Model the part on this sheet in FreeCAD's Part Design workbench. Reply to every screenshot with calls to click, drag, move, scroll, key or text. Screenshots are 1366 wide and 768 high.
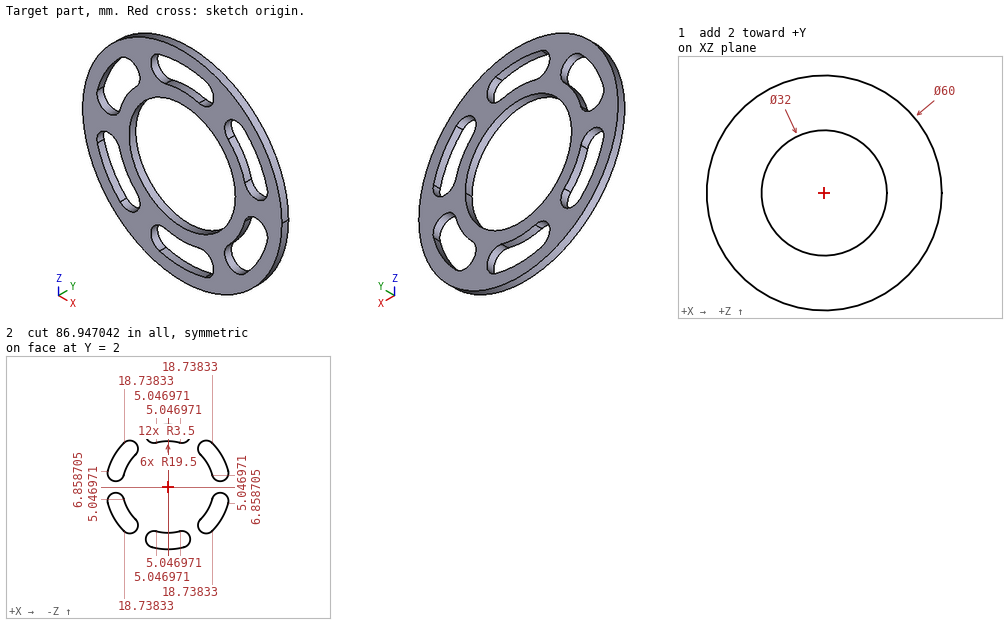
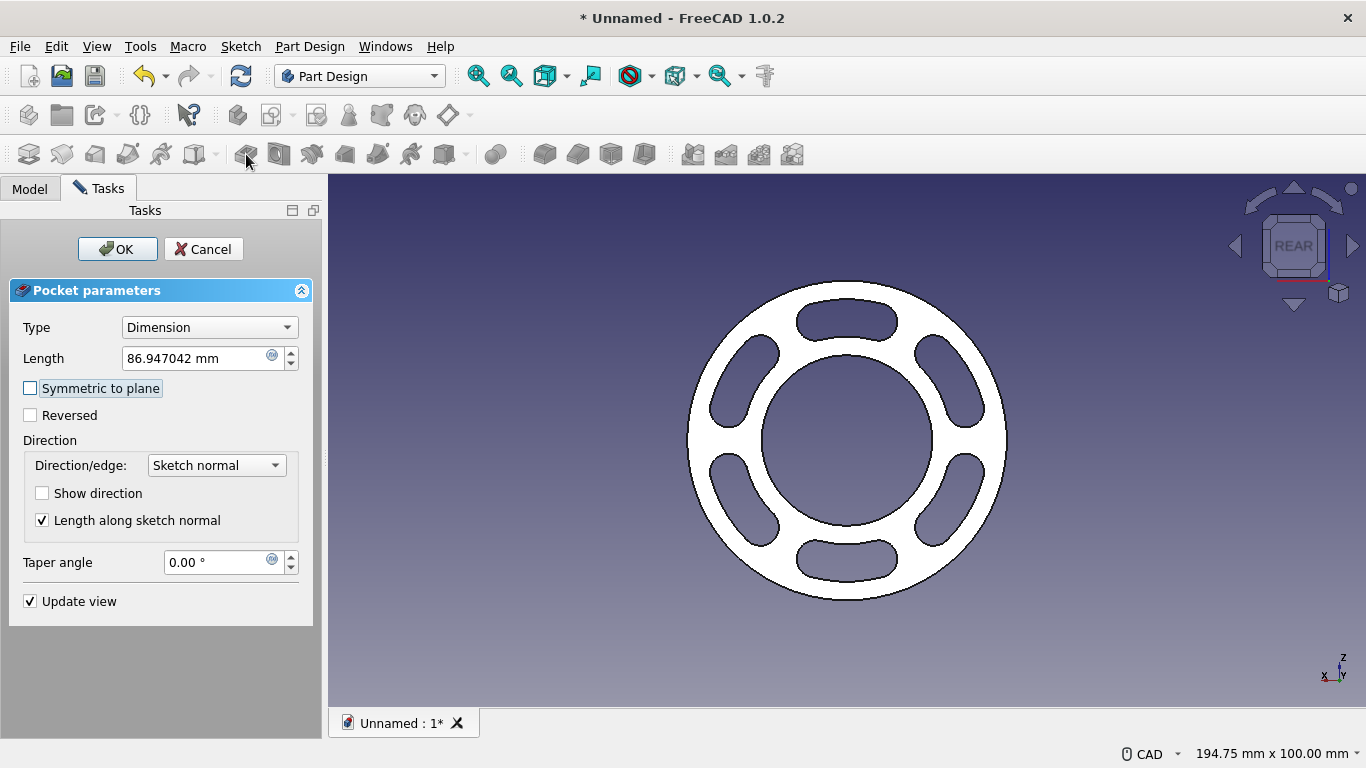
click(31, 388)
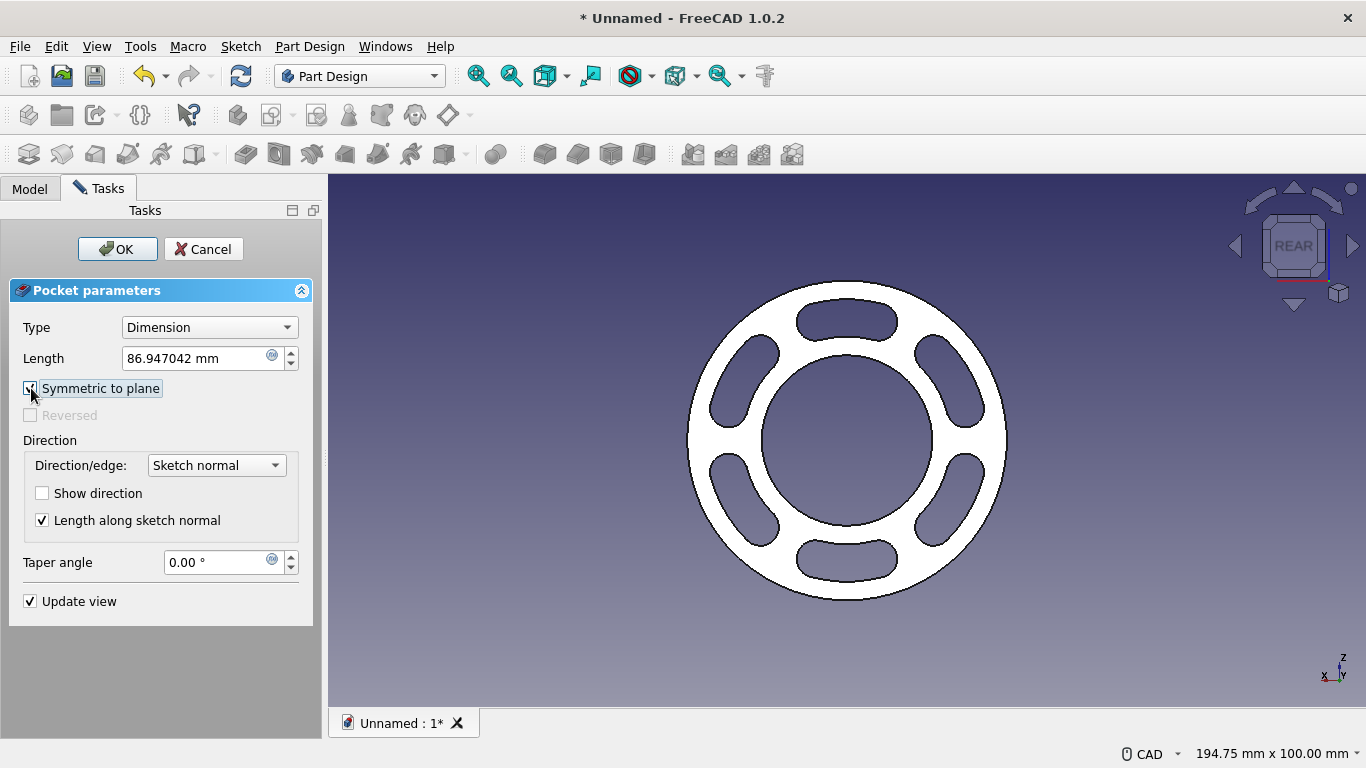
click(118, 249)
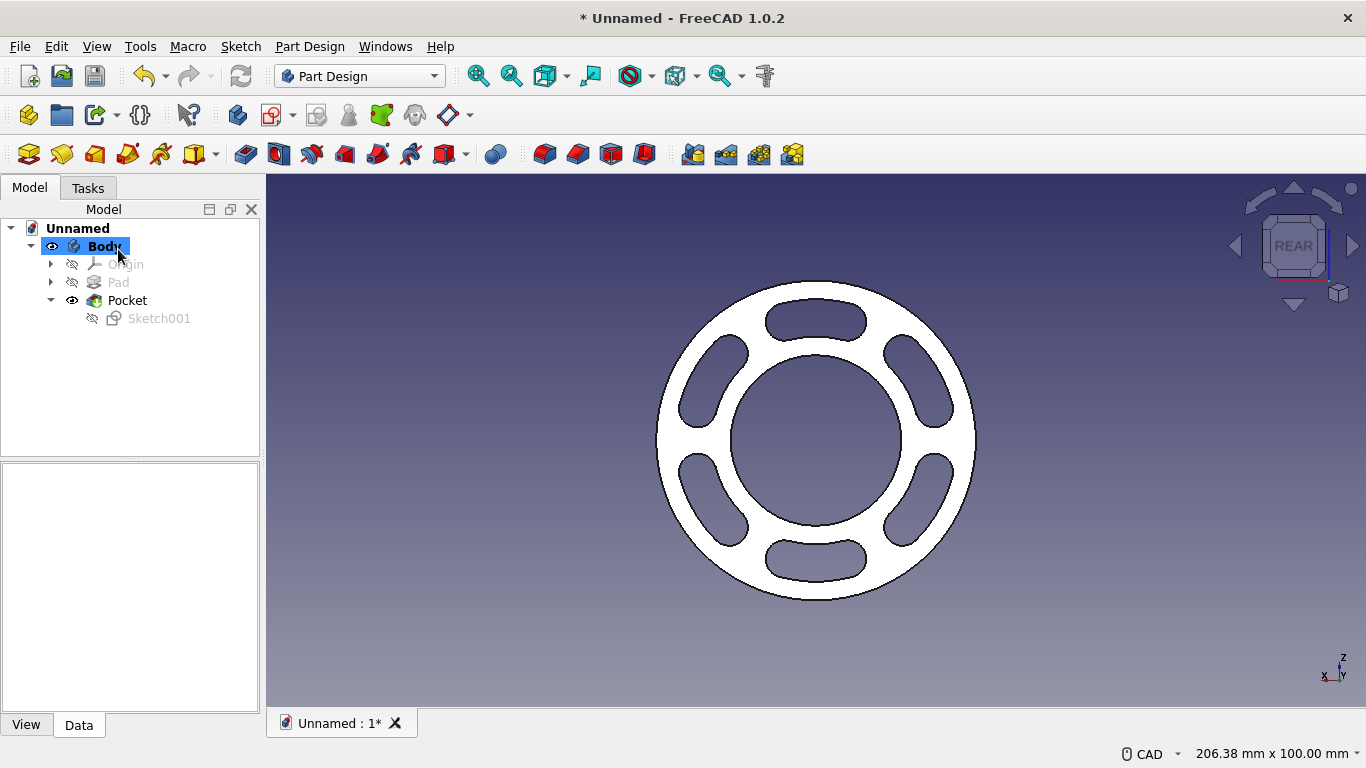
key(0)